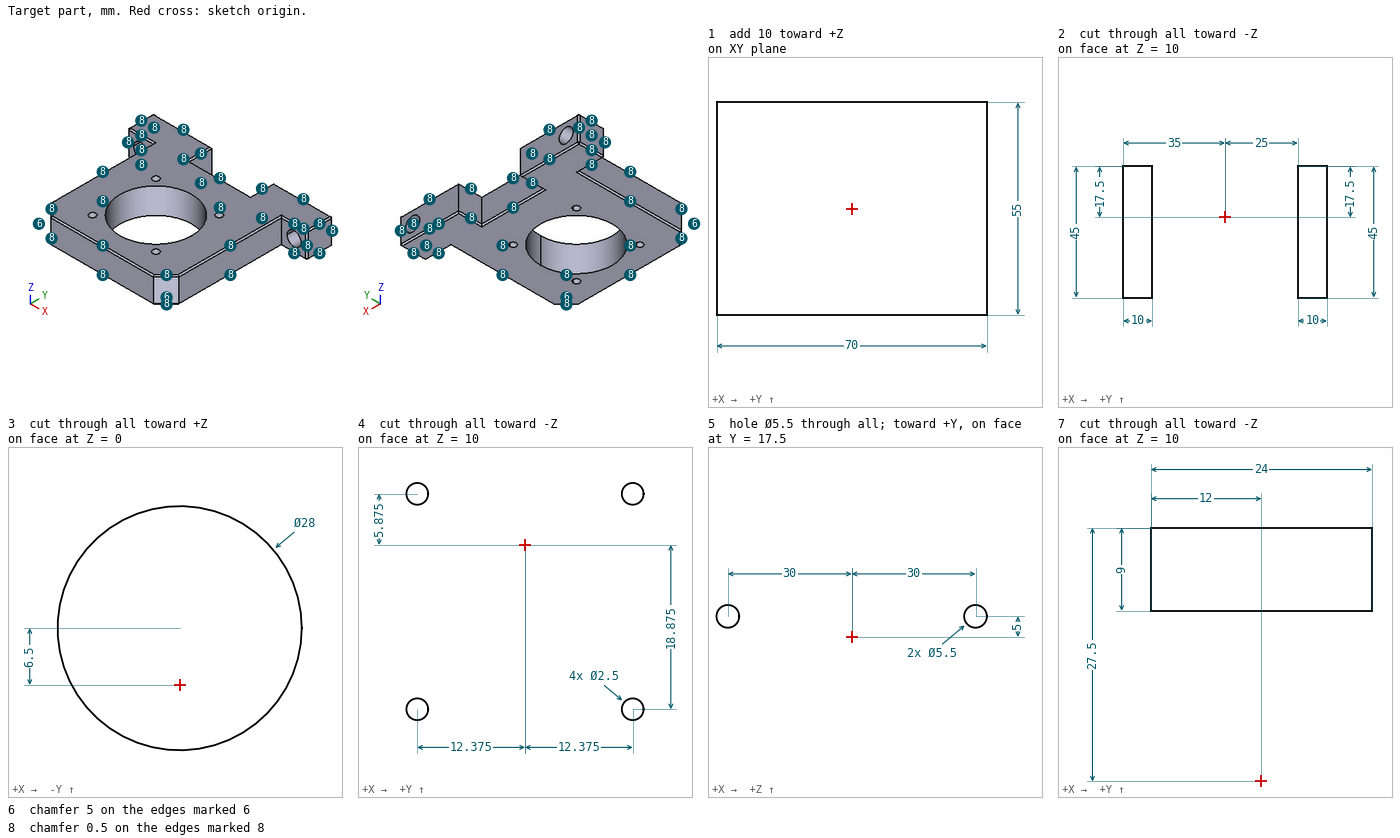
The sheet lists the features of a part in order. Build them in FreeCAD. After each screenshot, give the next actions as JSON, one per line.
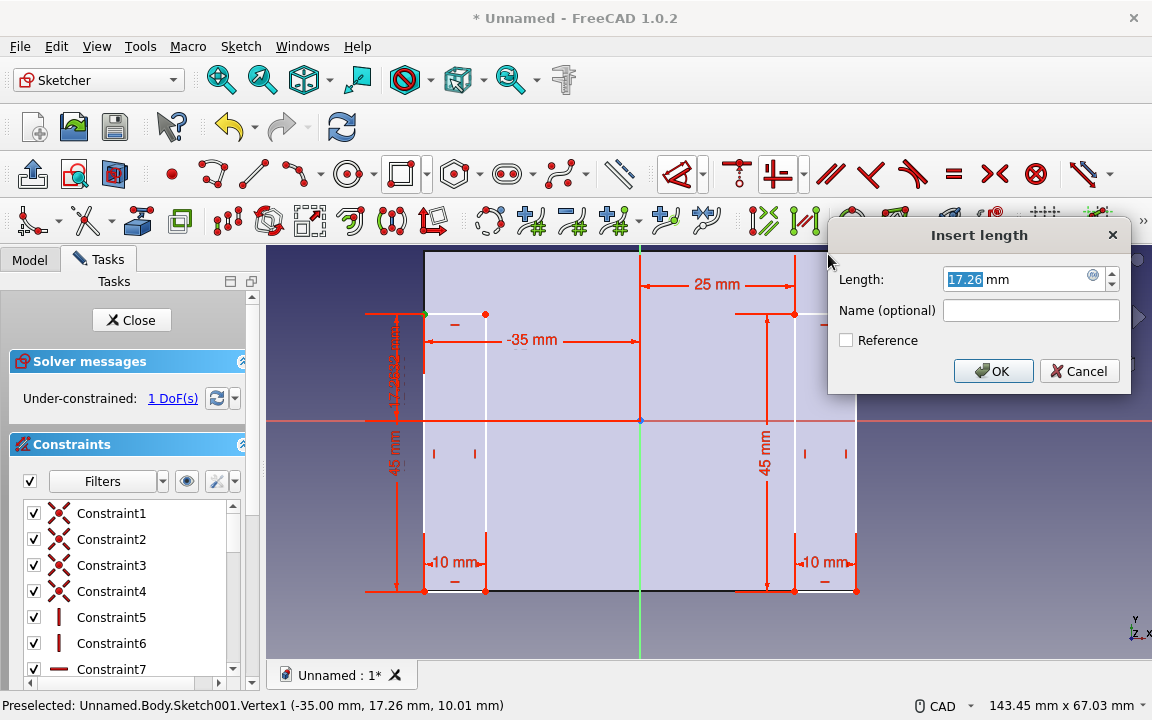
{"action": "type", "text": "17.5"}
{"action": "key", "text": "Return"}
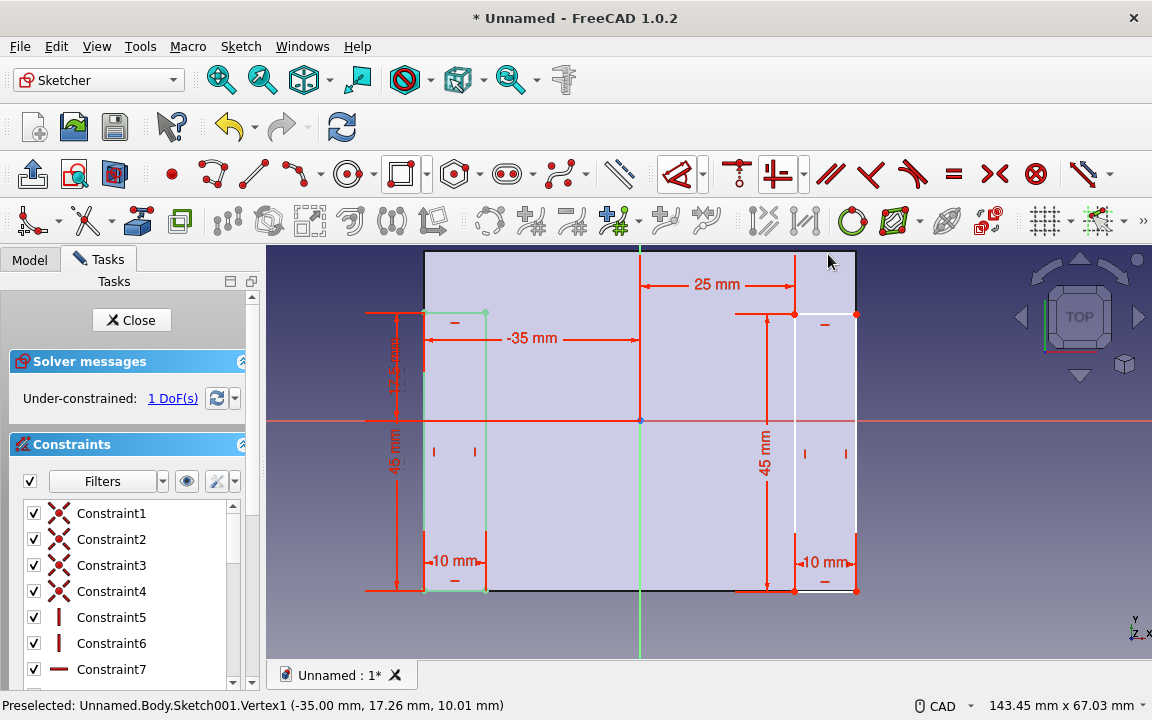
{"action": "left_click", "coordinate": [795, 314]}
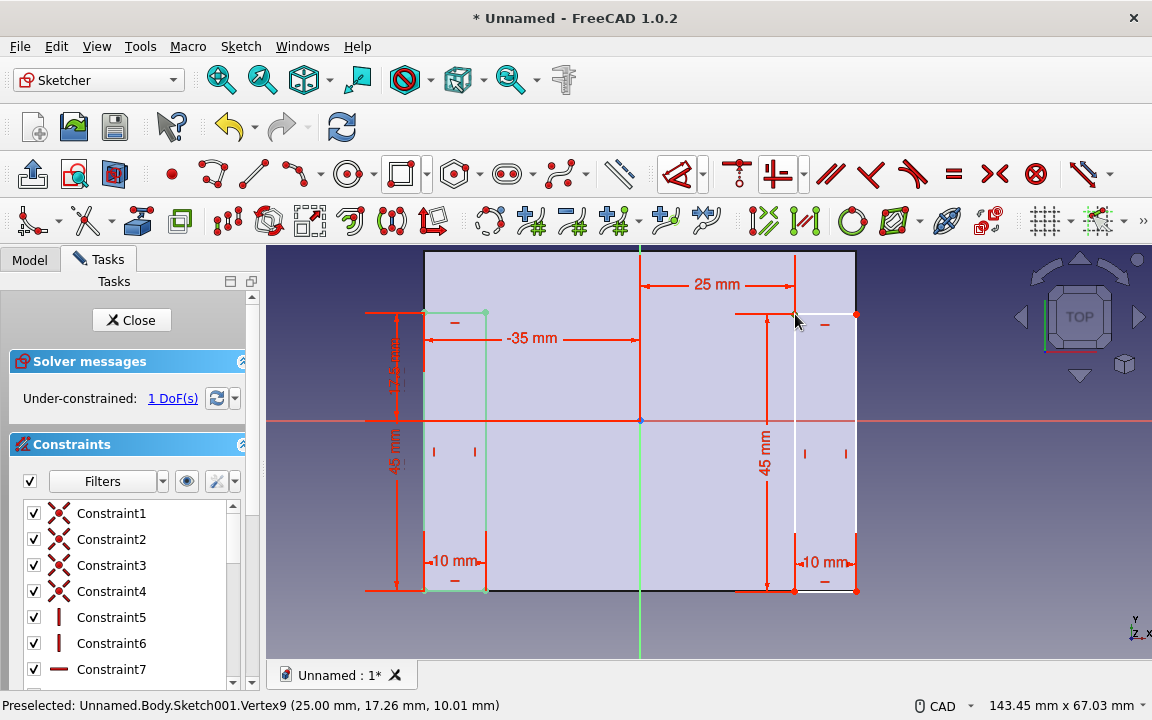
{"action": "key", "text": "i"}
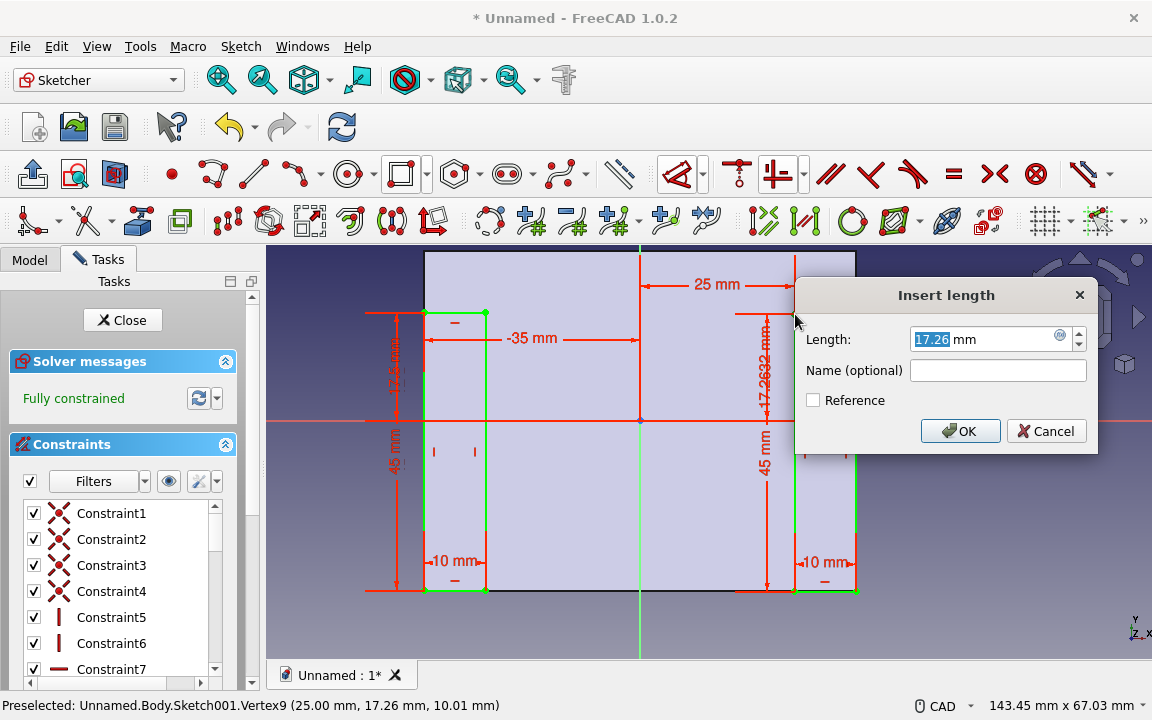
{"action": "type", "text": "17.5"}
{"action": "key", "text": "Return"}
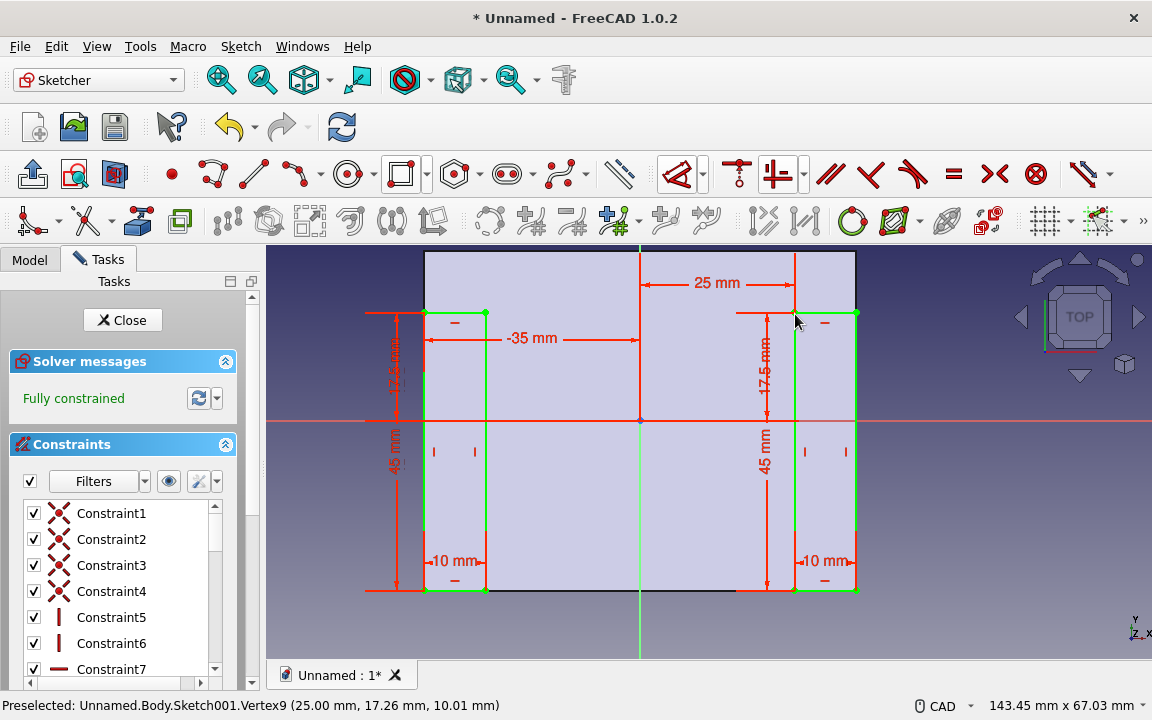
{"action": "left_click", "coordinate": [123, 320]}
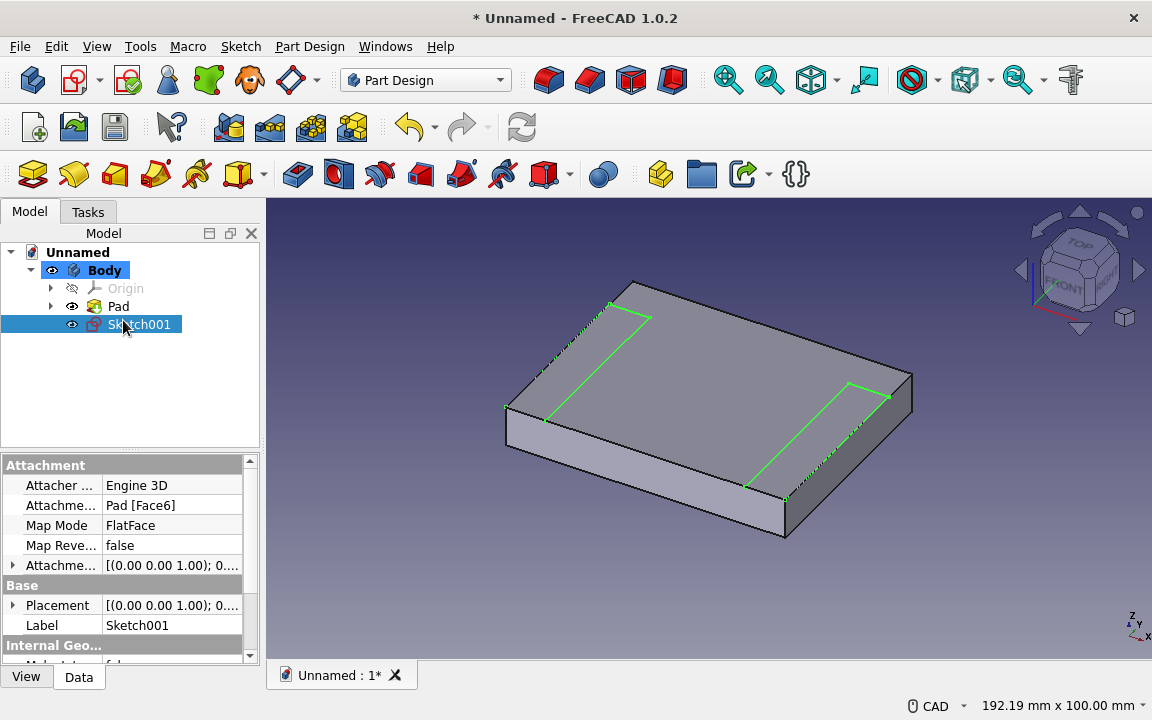
{"action": "left_click", "coordinate": [298, 174]}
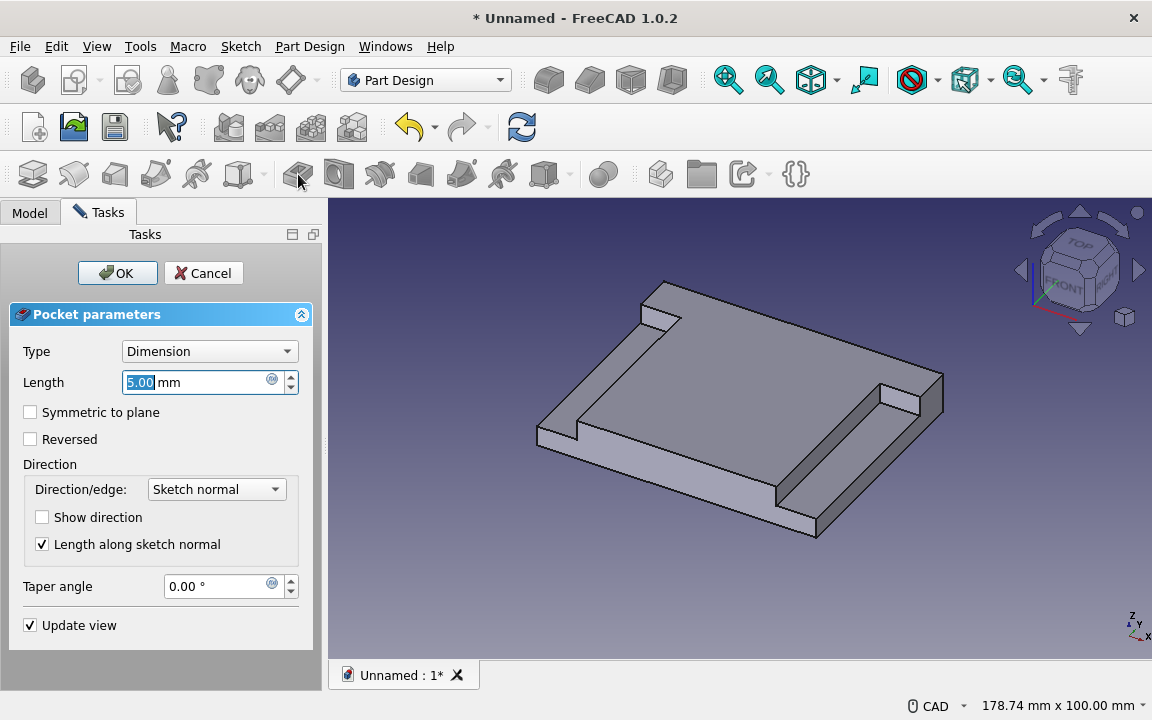
{"action": "left_click", "coordinate": [210, 352]}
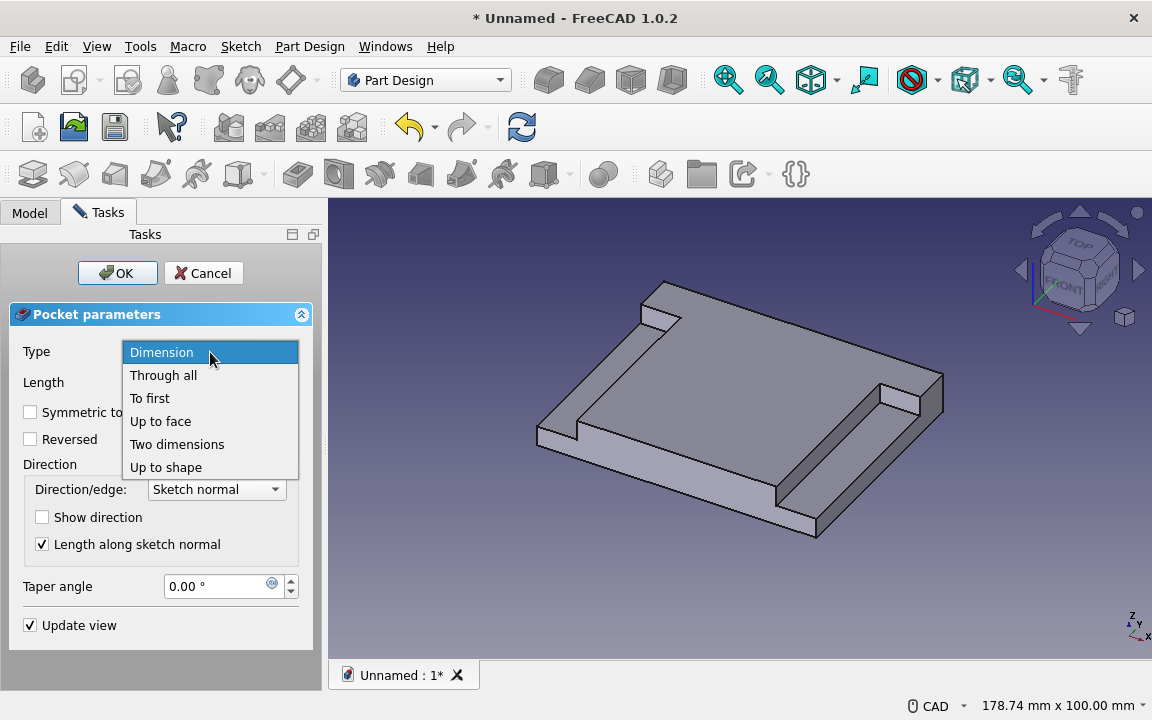
{"action": "left_click", "coordinate": [208, 376]}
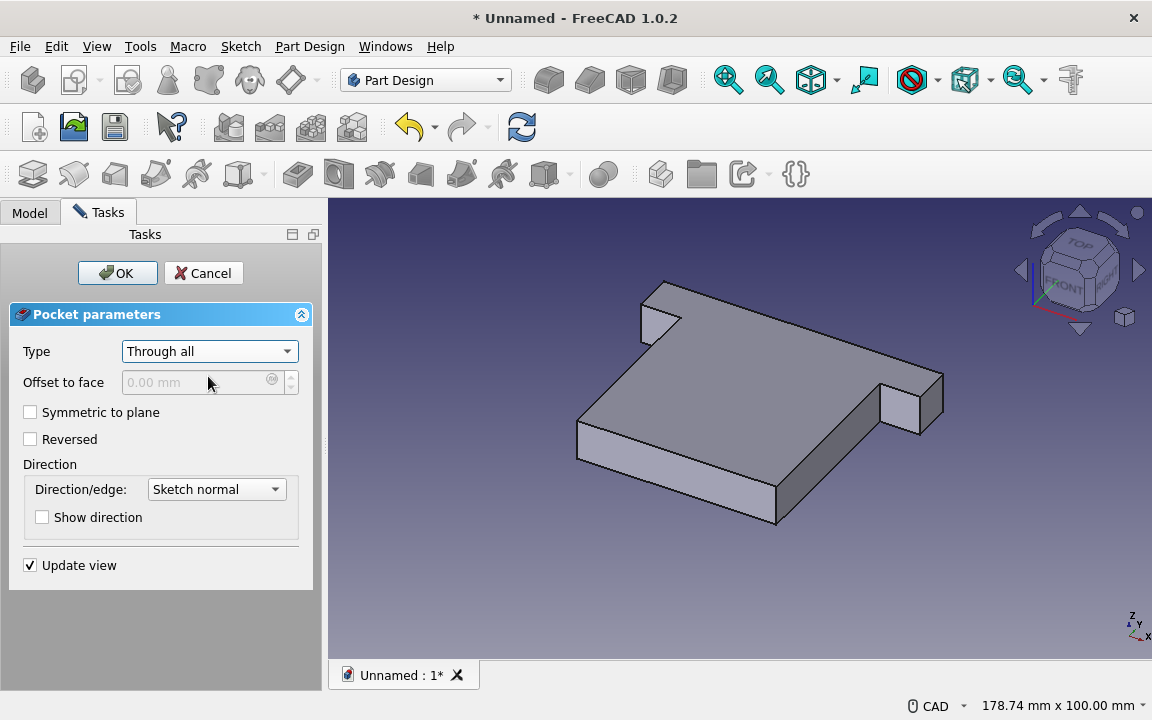
{"action": "left_click", "coordinate": [118, 273]}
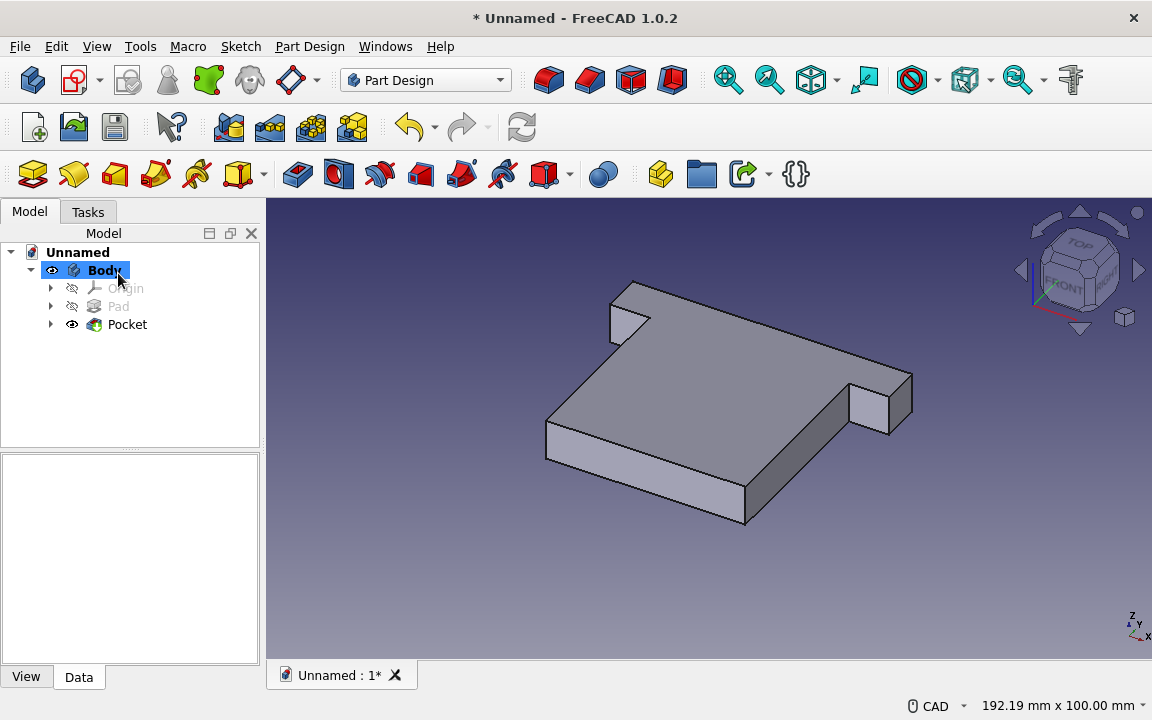
{"action": "key", "text": "5"}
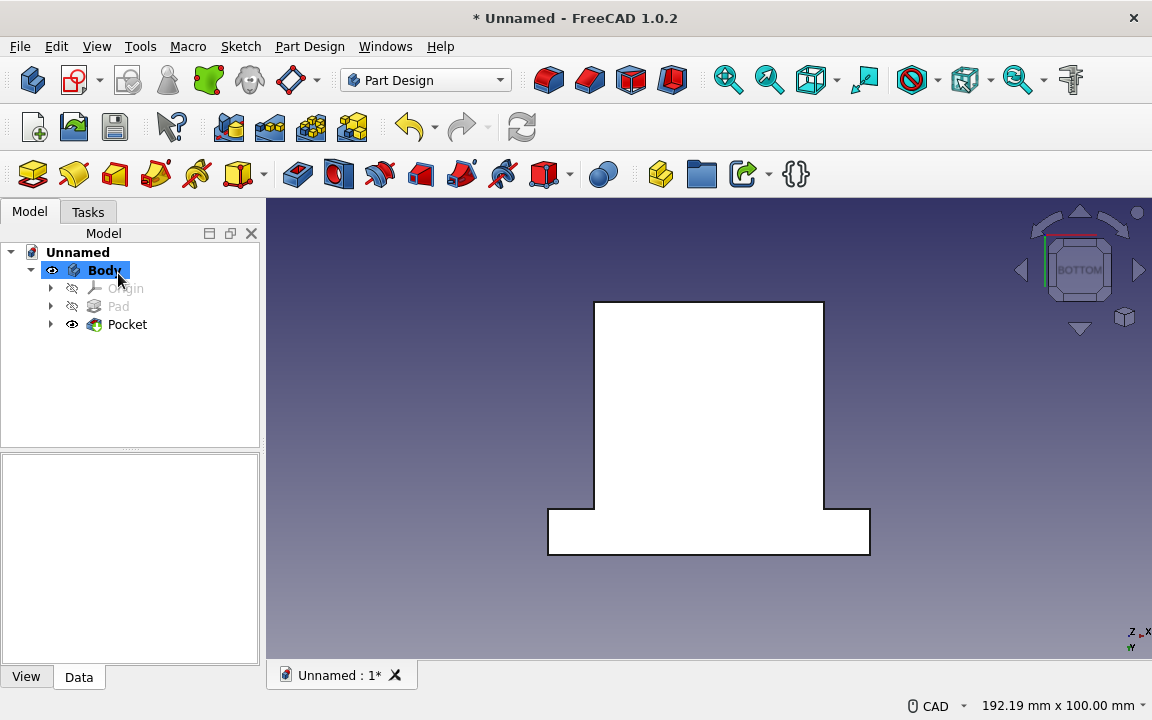
{"action": "left_click", "coordinate": [709, 427]}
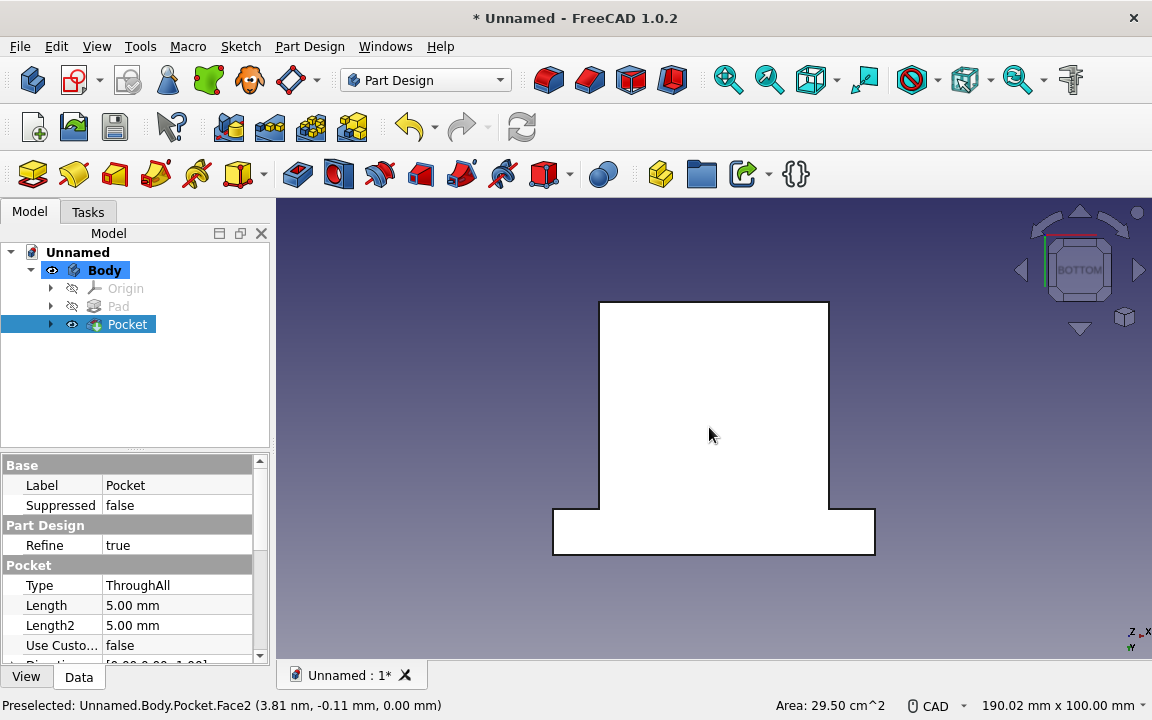
{"action": "left_click", "coordinate": [74, 80]}